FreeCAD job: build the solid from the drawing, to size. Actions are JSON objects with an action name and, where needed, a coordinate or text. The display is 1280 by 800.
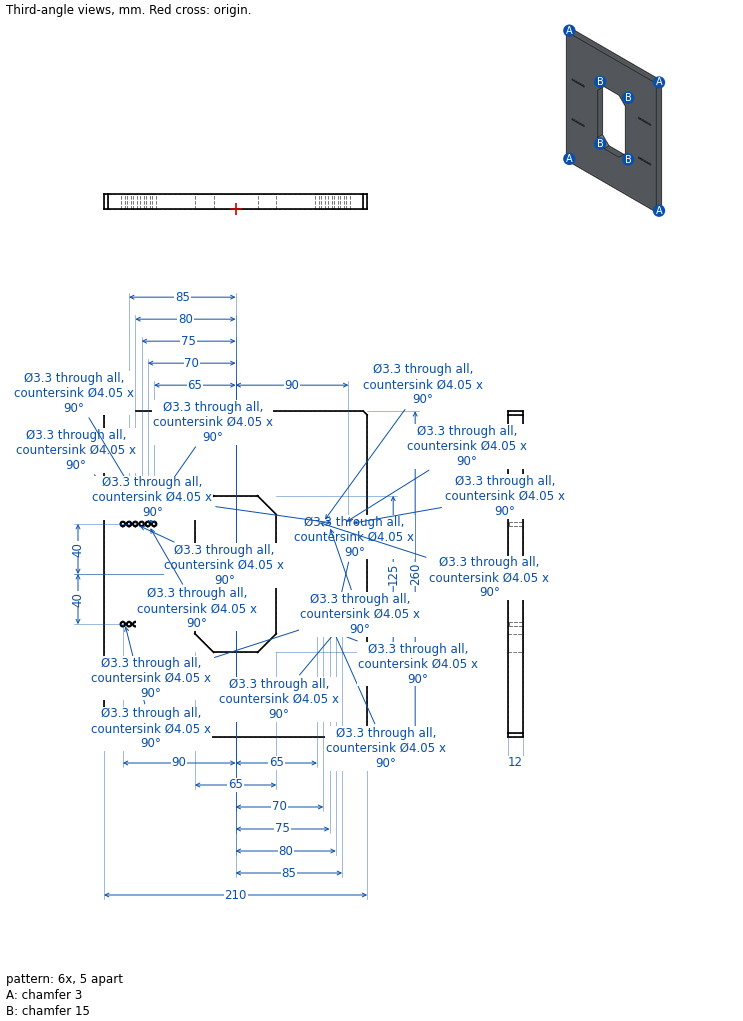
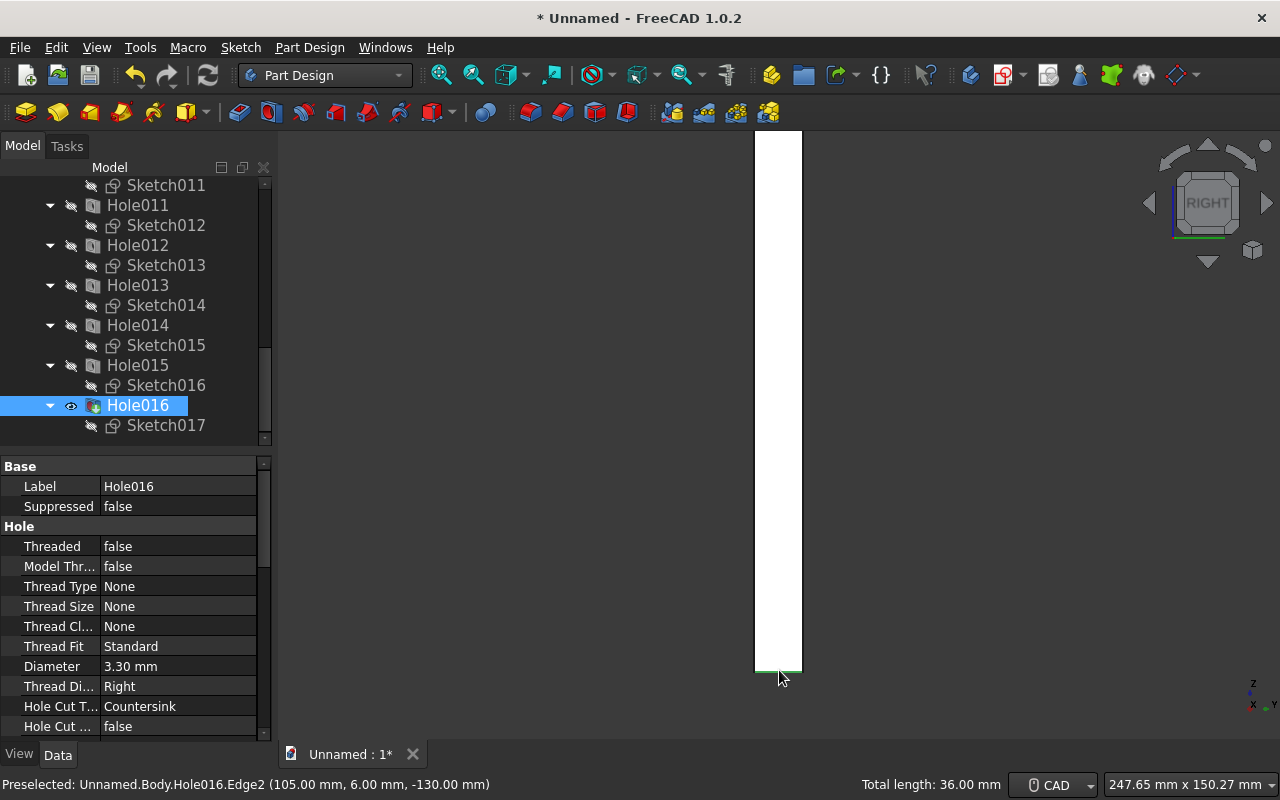
{"action": "left_click", "coordinate": [442, 76]}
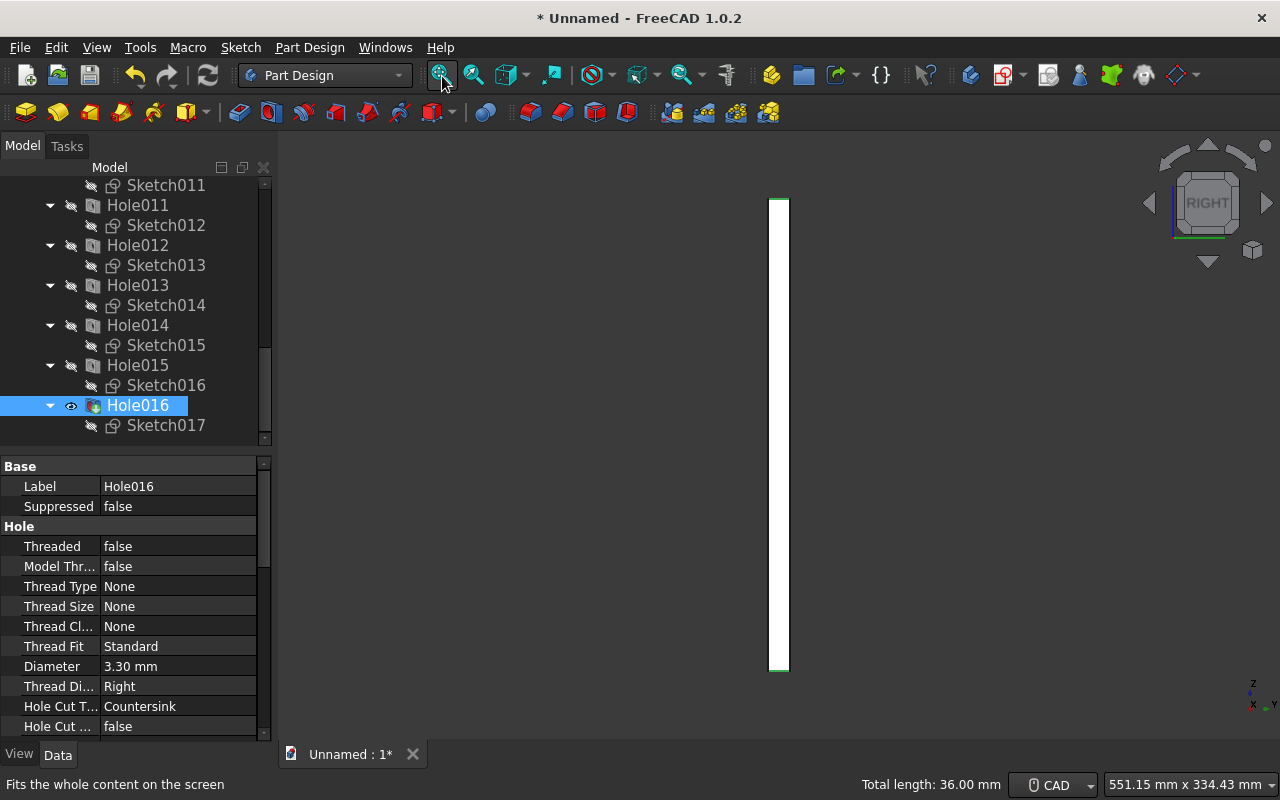
{"action": "key", "text": "5"}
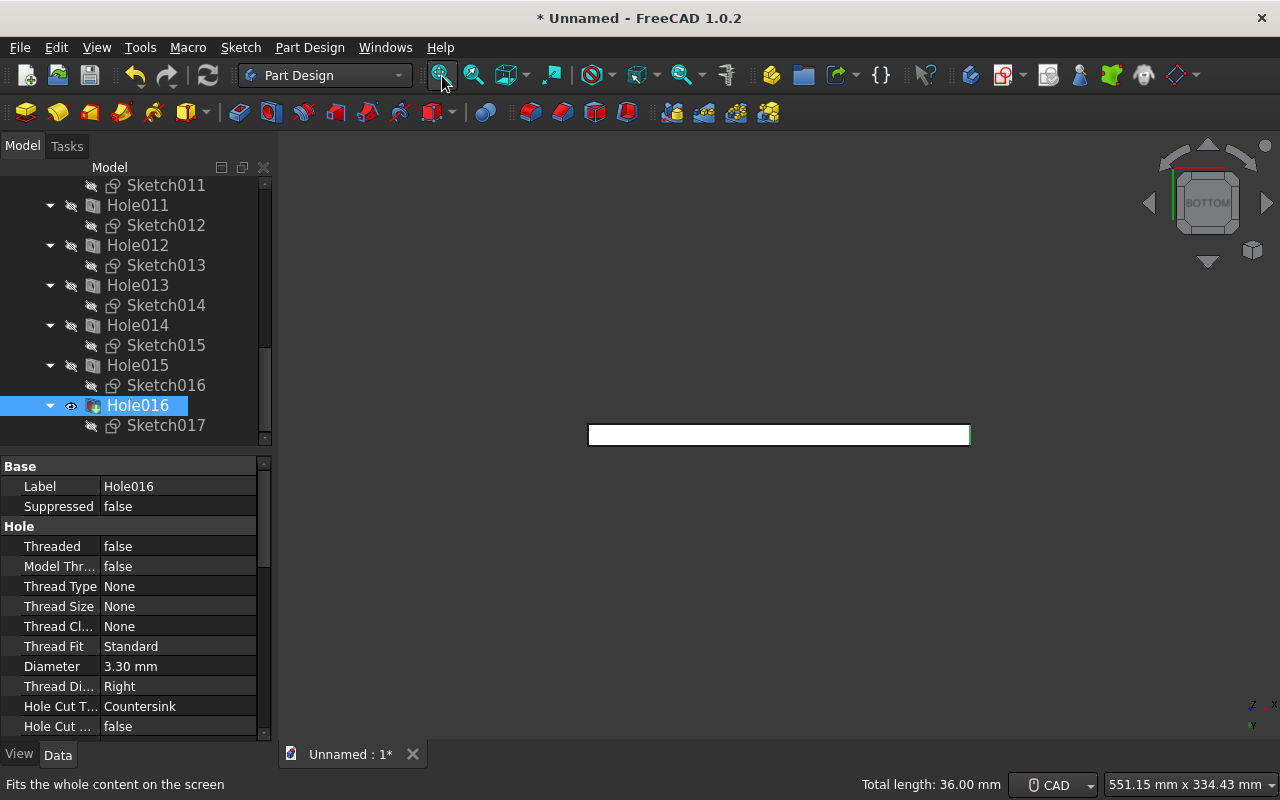
{"action": "left_click", "coordinate": [442, 76]}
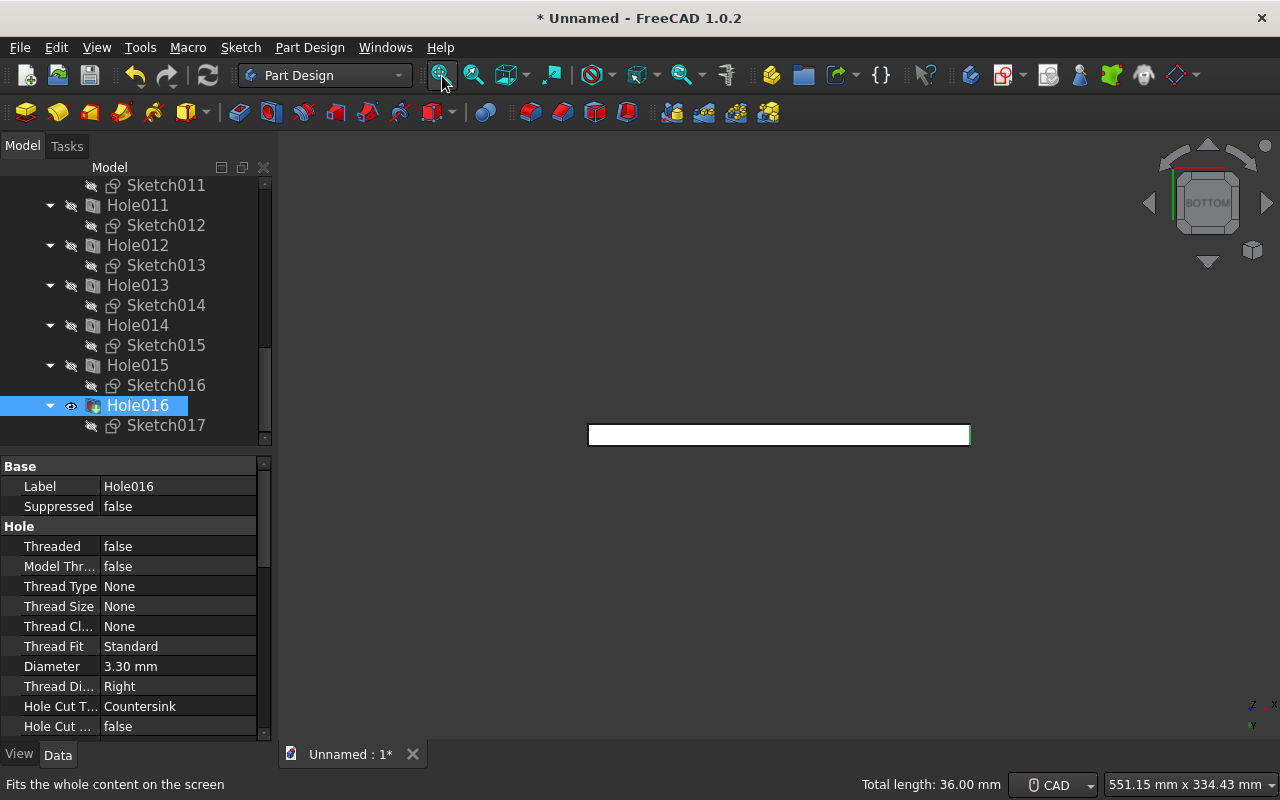
{"action": "left_click", "coordinate": [588, 434], "text": "ctrl"}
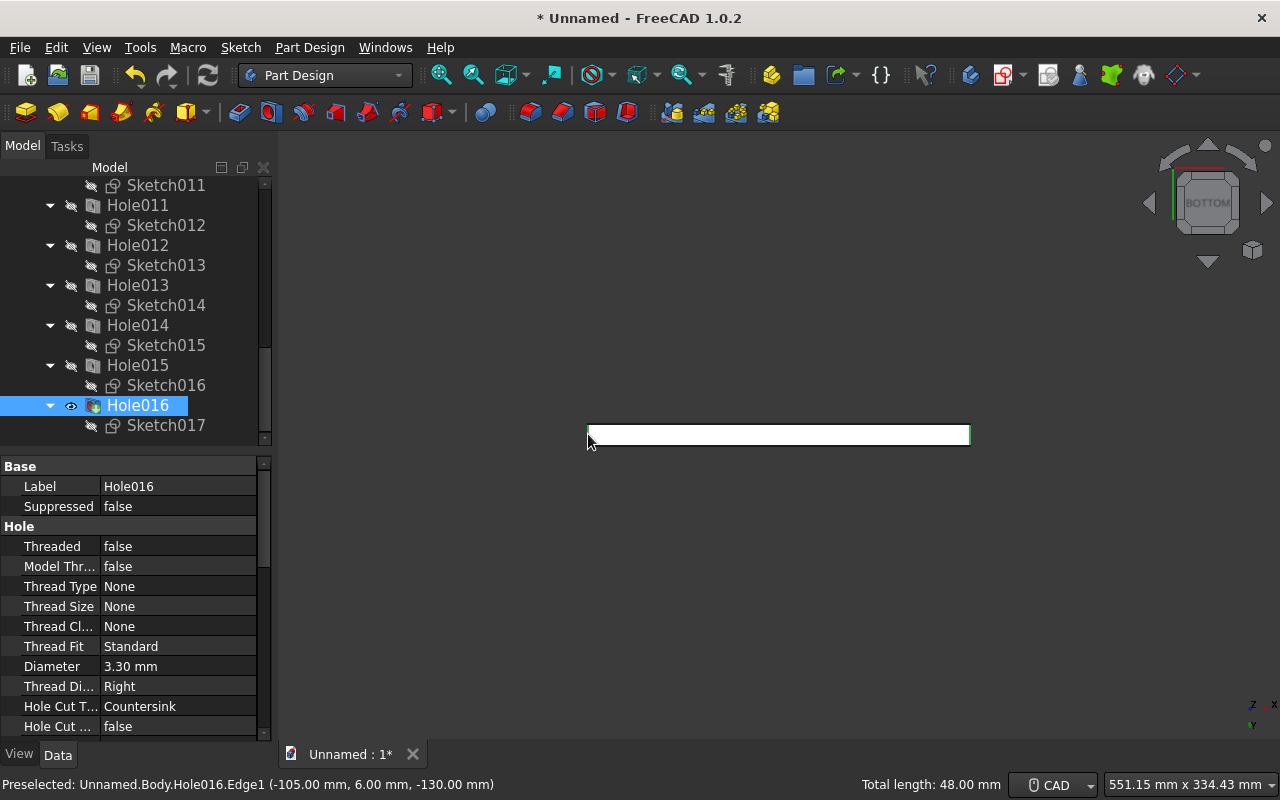
{"action": "left_click", "coordinate": [564, 112]}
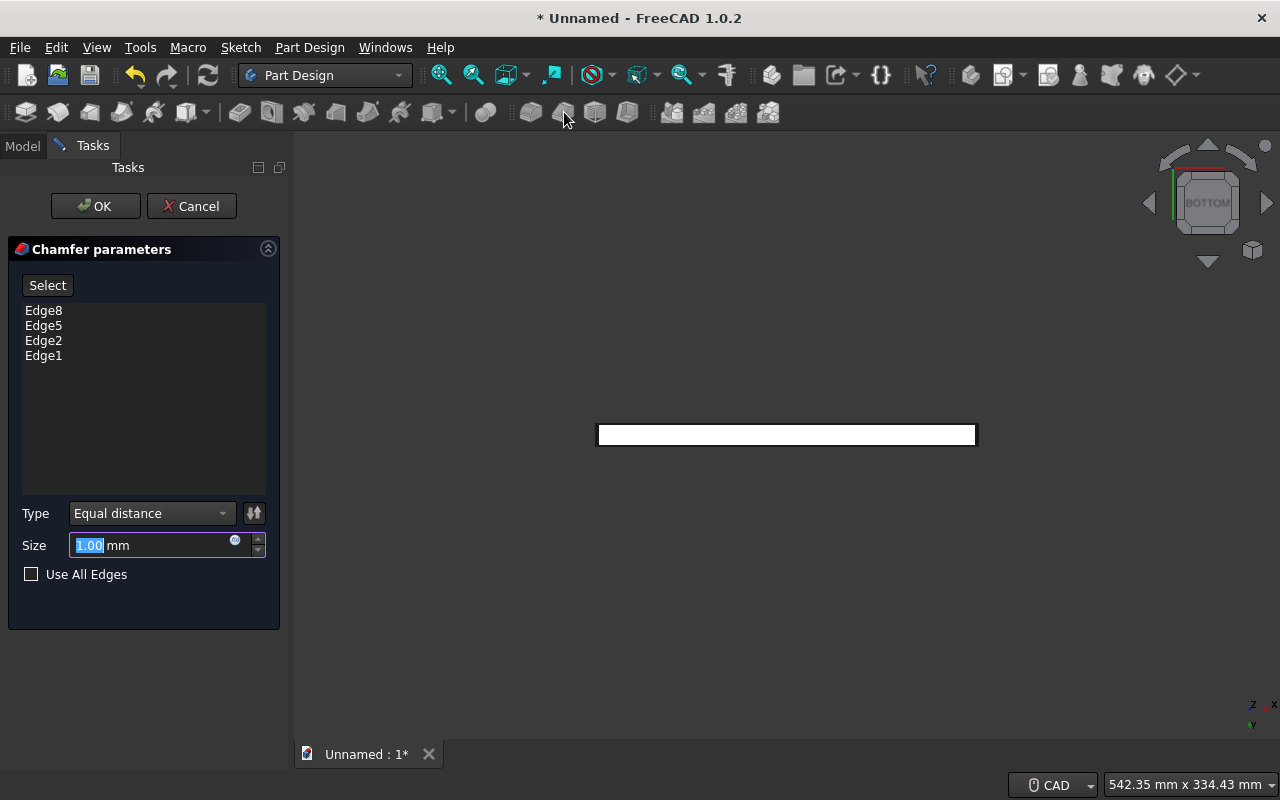
{"action": "type", "text": "3"}
{"action": "key", "text": "Tab"}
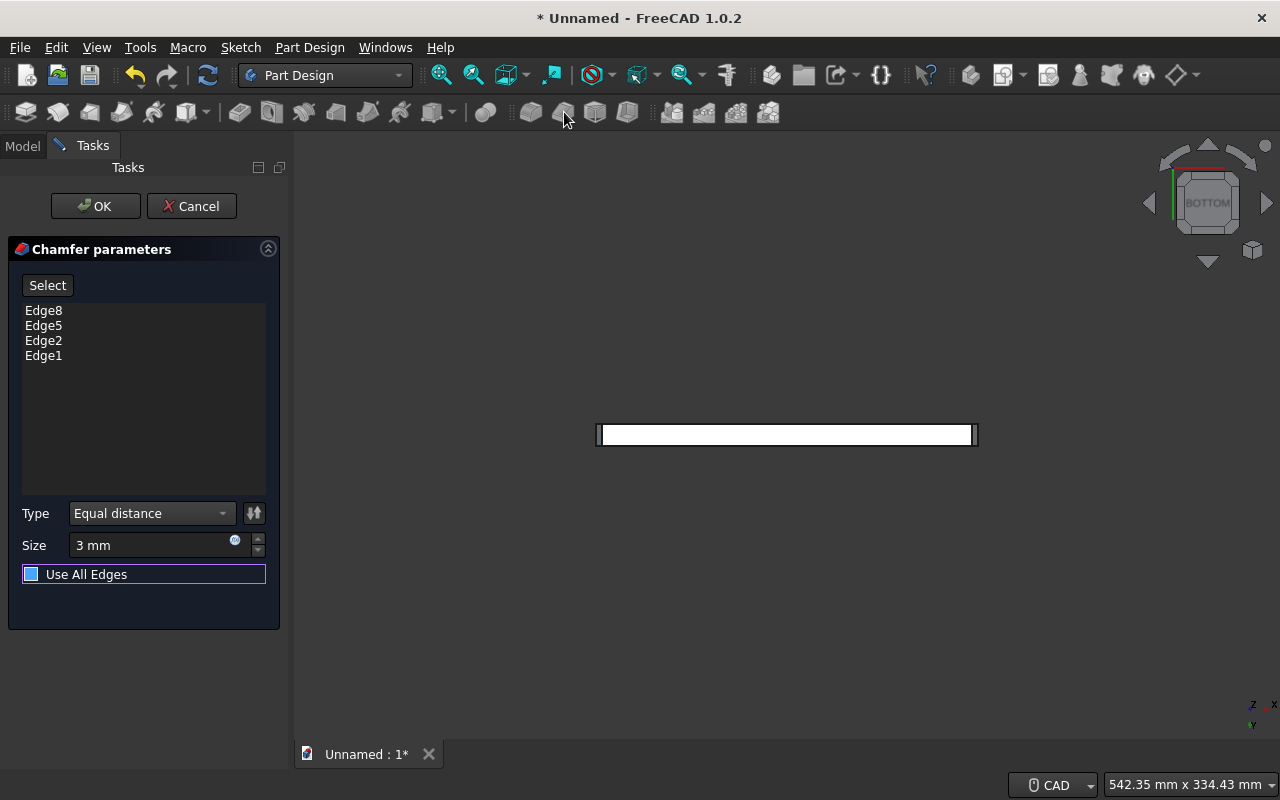
{"action": "left_click", "coordinate": [96, 206]}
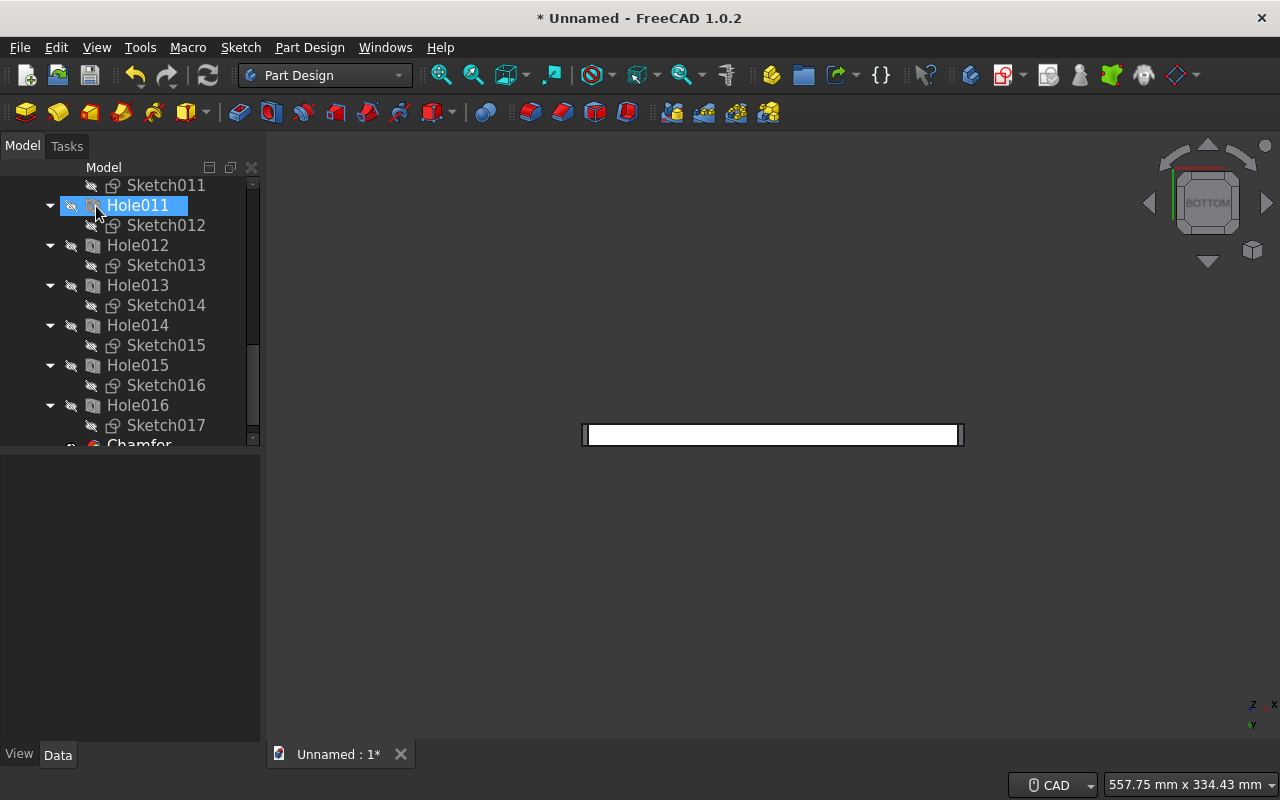
{"action": "left_click", "coordinate": [442, 76]}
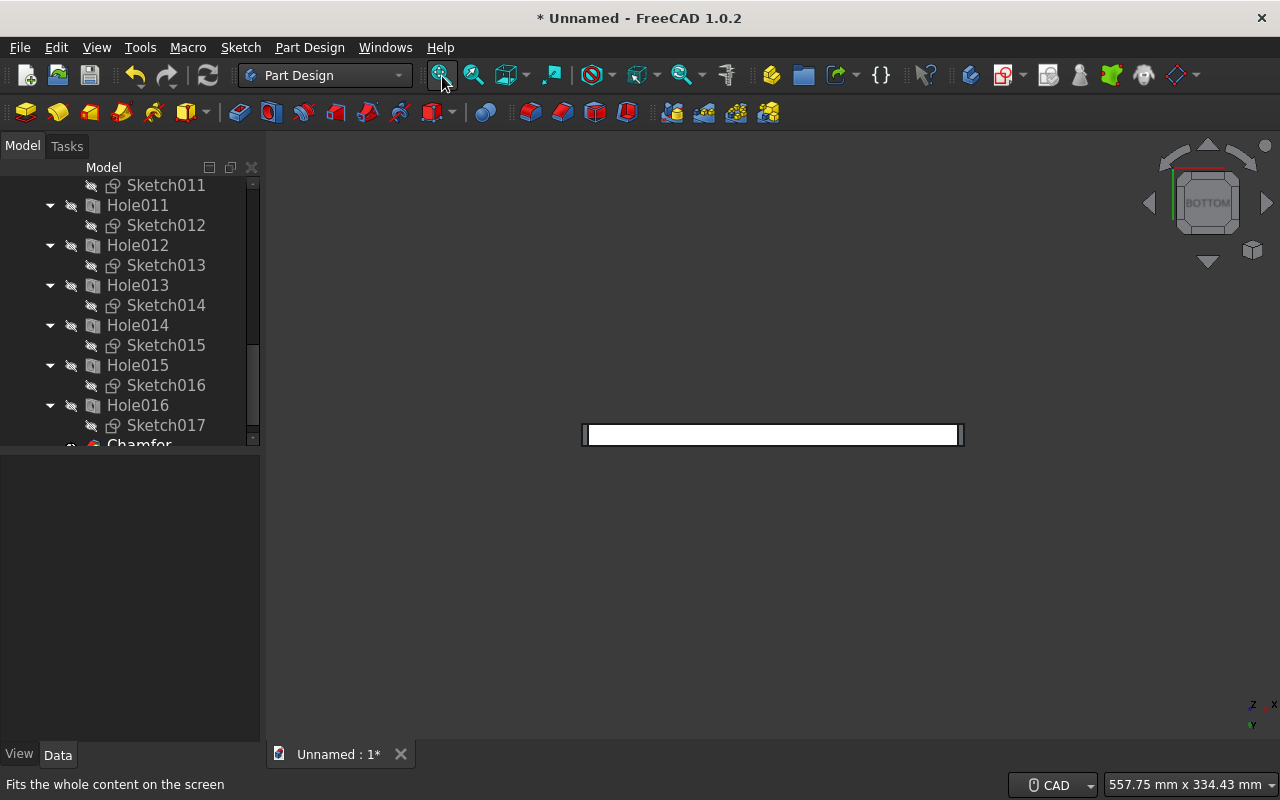
{"action": "key", "text": "0"}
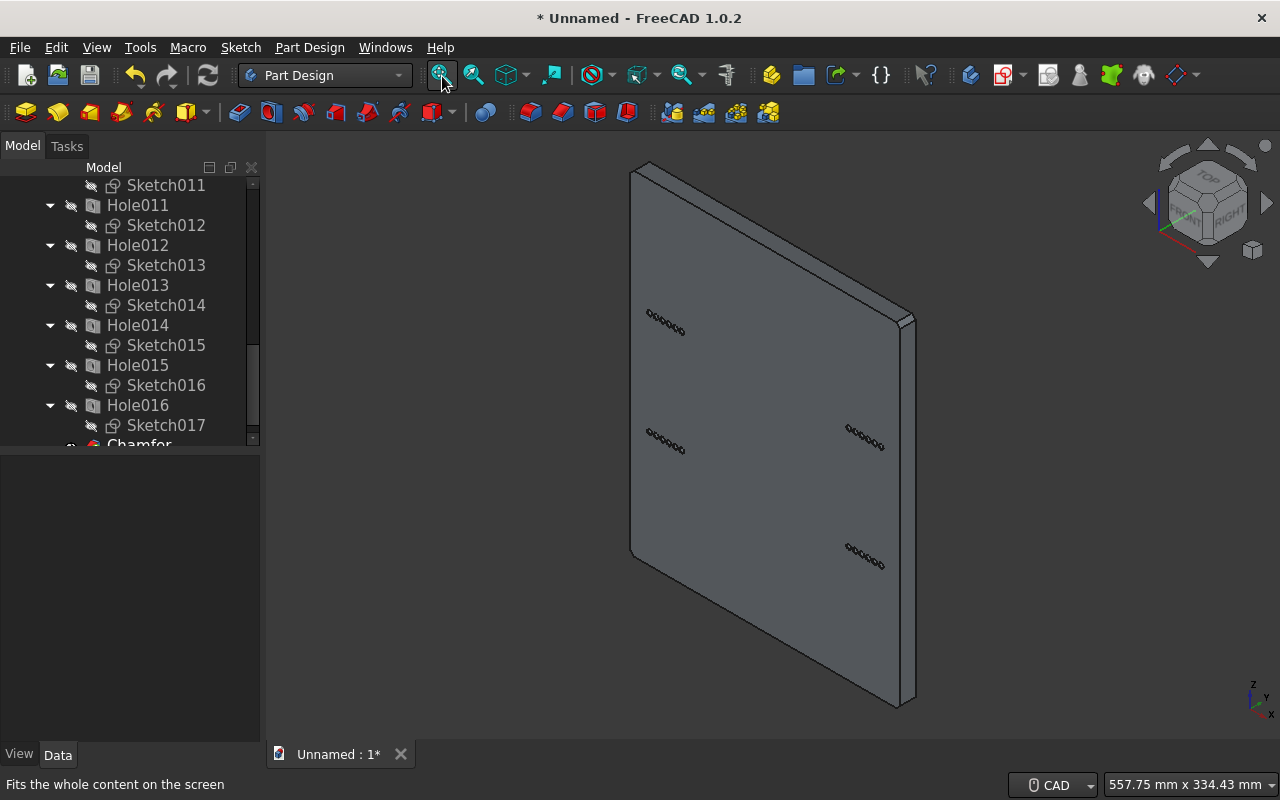
{"action": "left_click", "coordinate": [765, 438]}